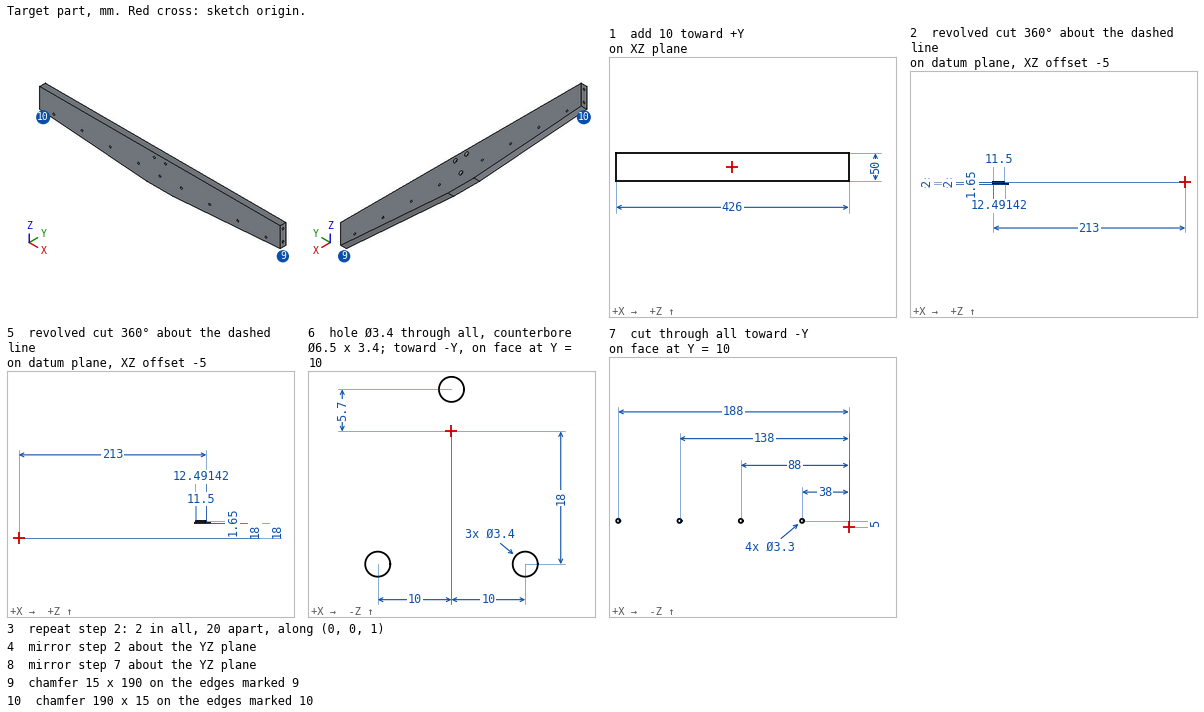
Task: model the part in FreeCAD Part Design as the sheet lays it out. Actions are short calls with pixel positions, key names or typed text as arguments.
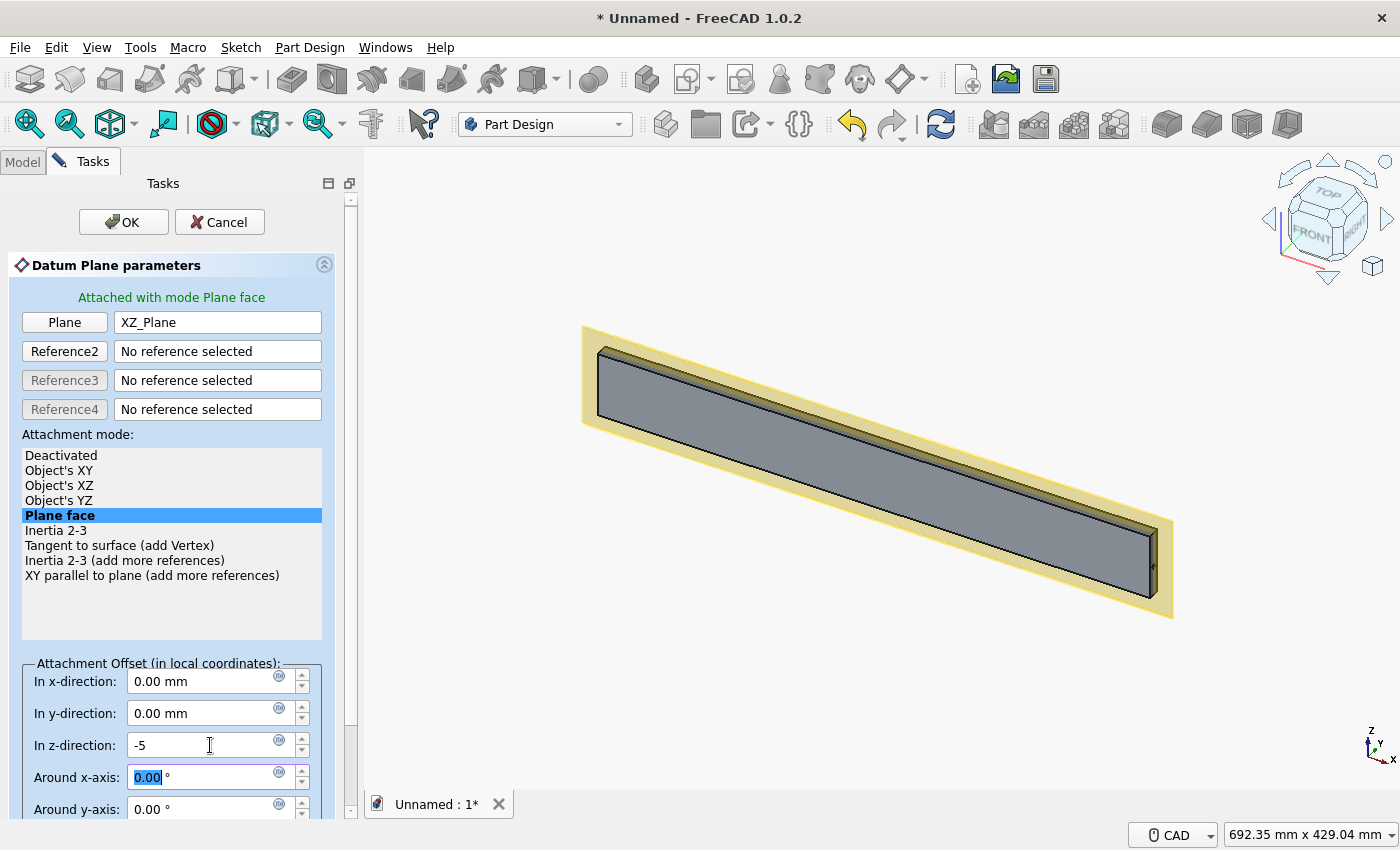
click(124, 222)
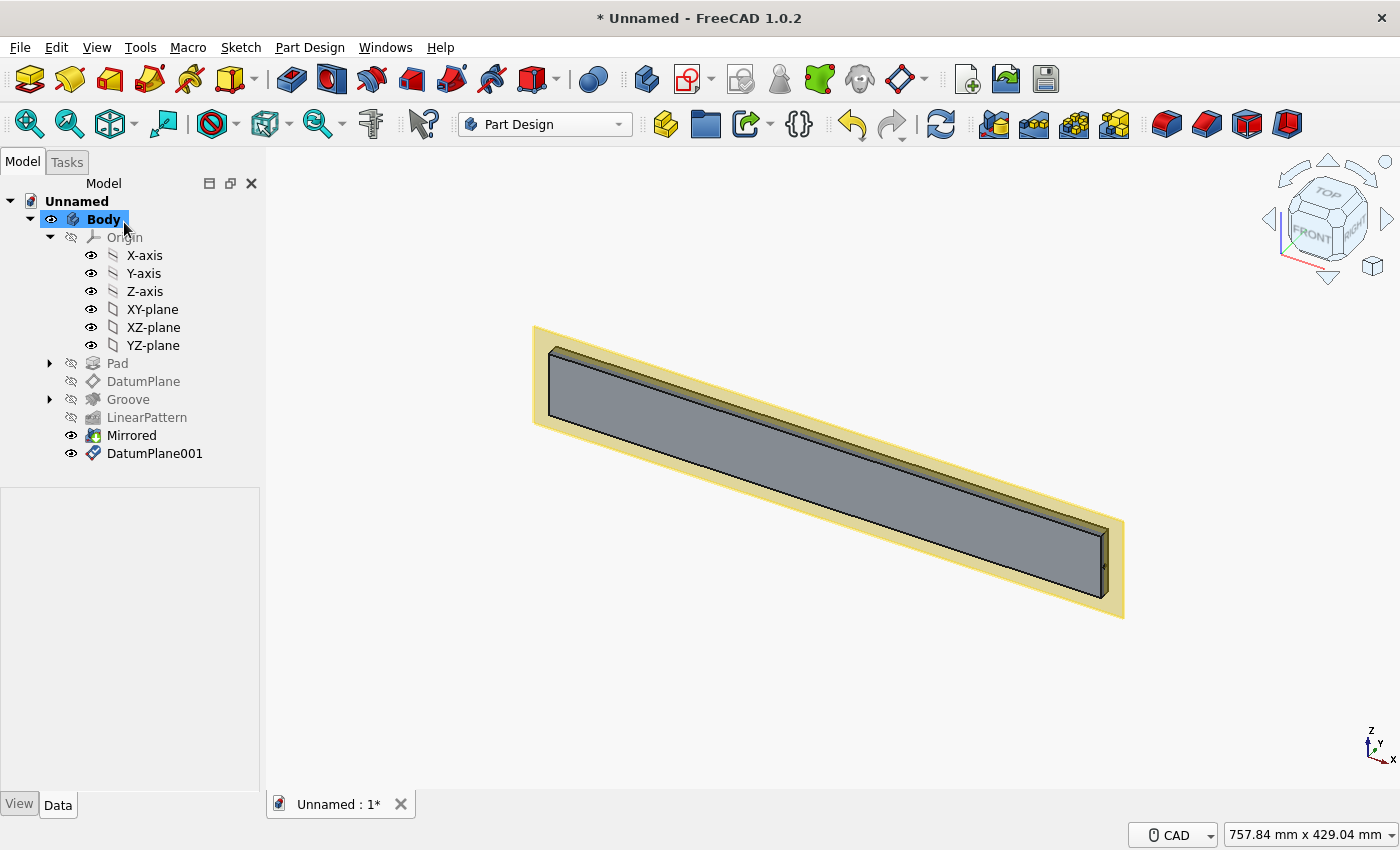
click(116, 453)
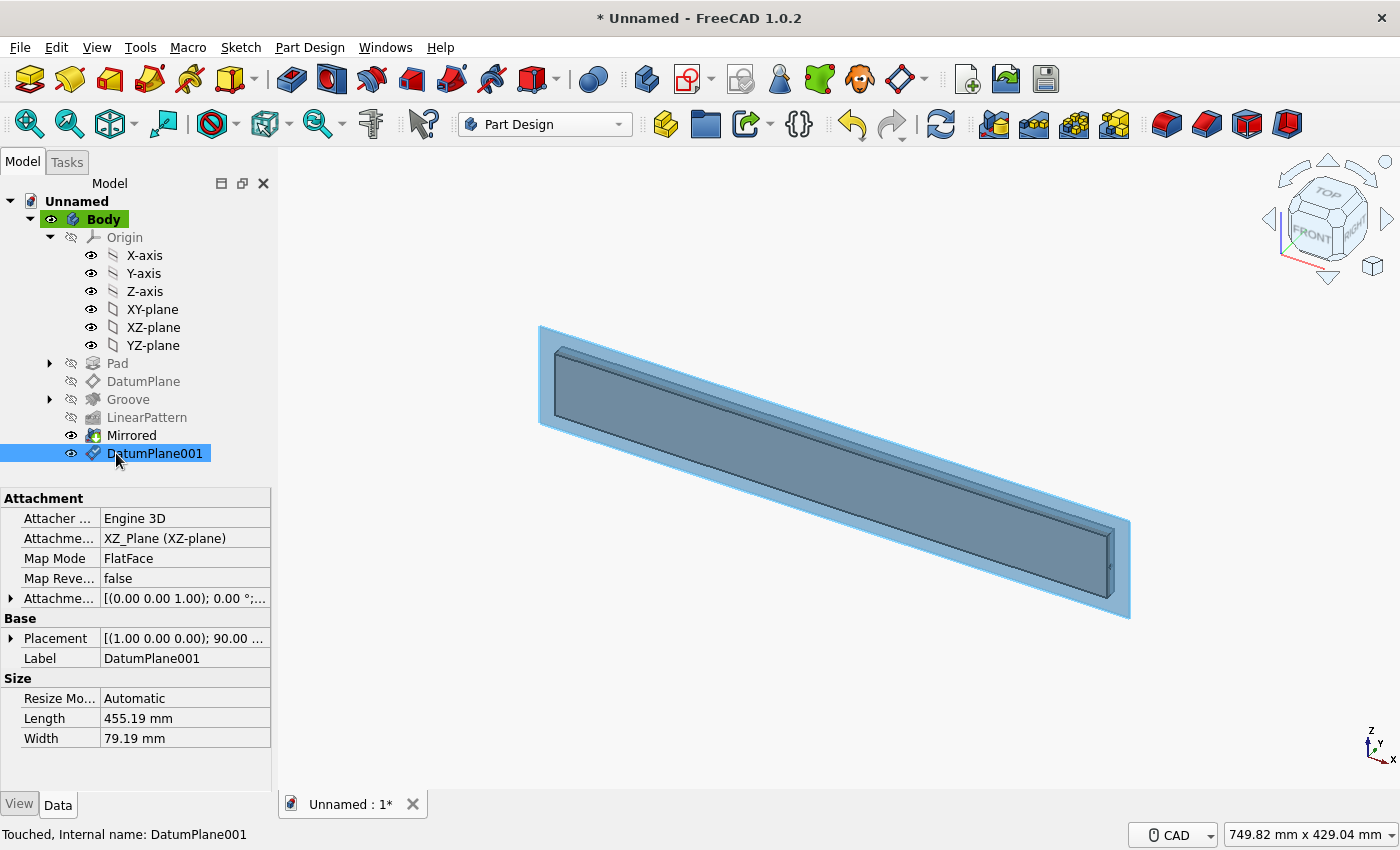
click(688, 80)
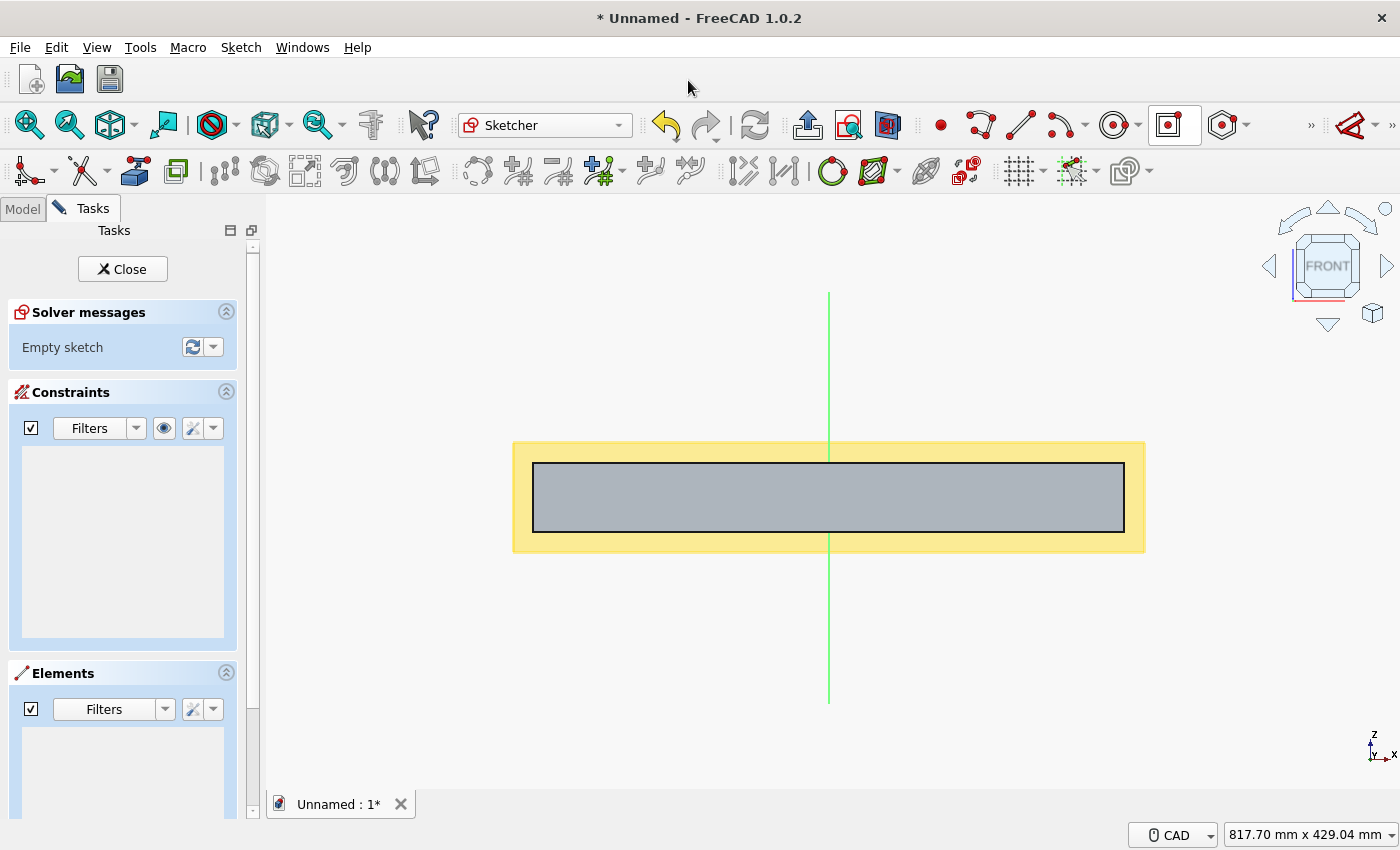
key(q)
key(s)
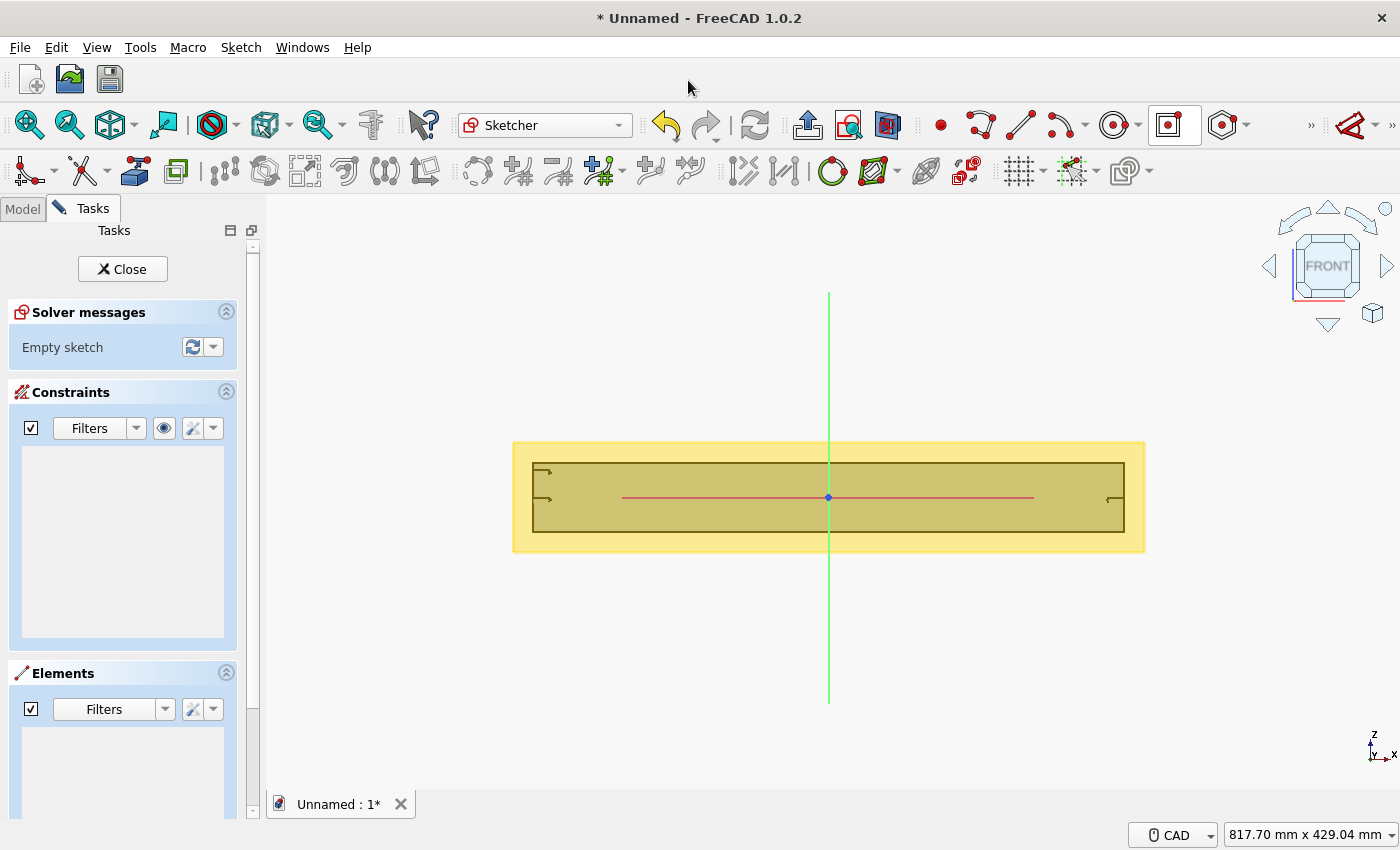
scroll(1137, 470, up, 15)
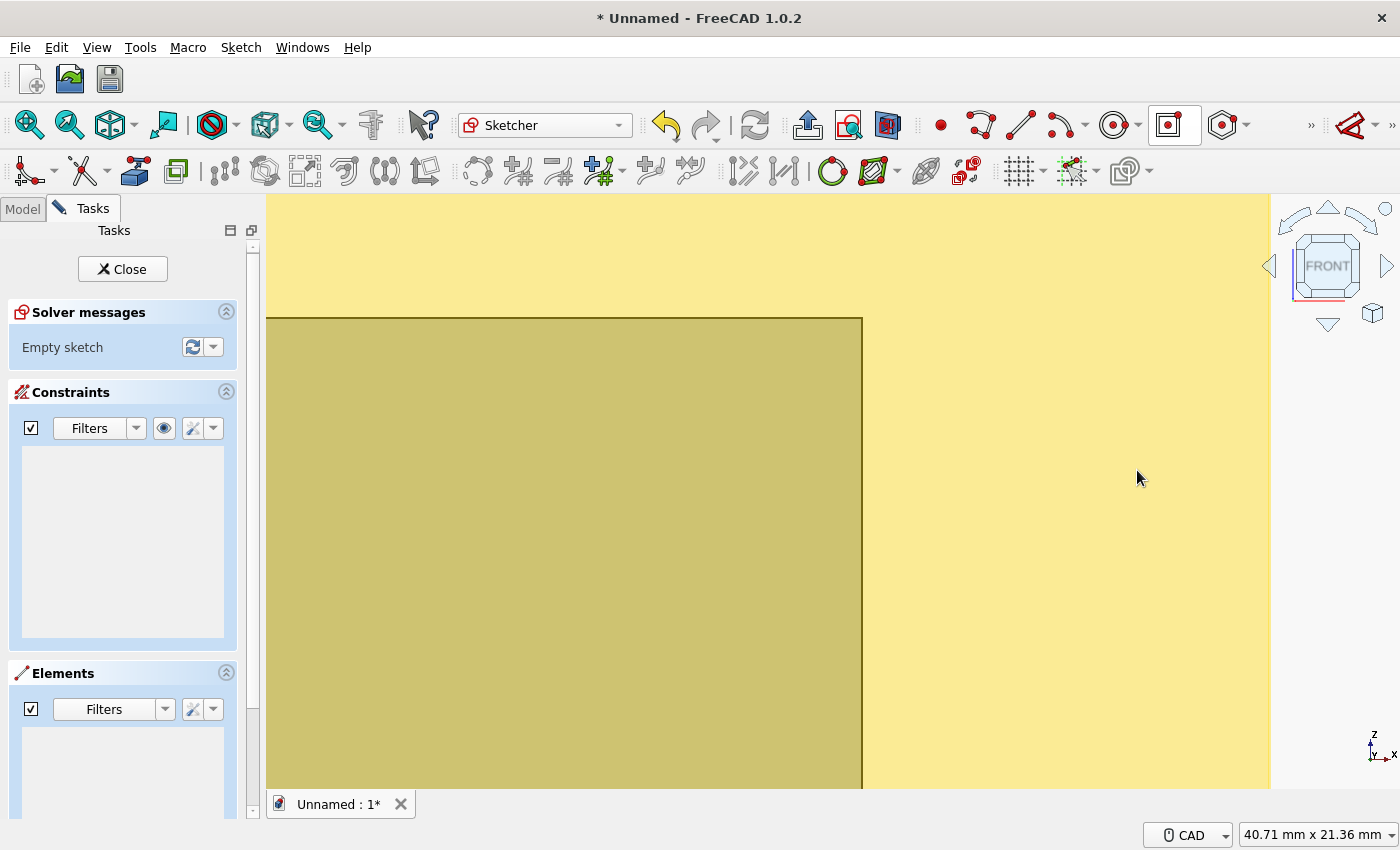
scroll(745, 488, up, 2)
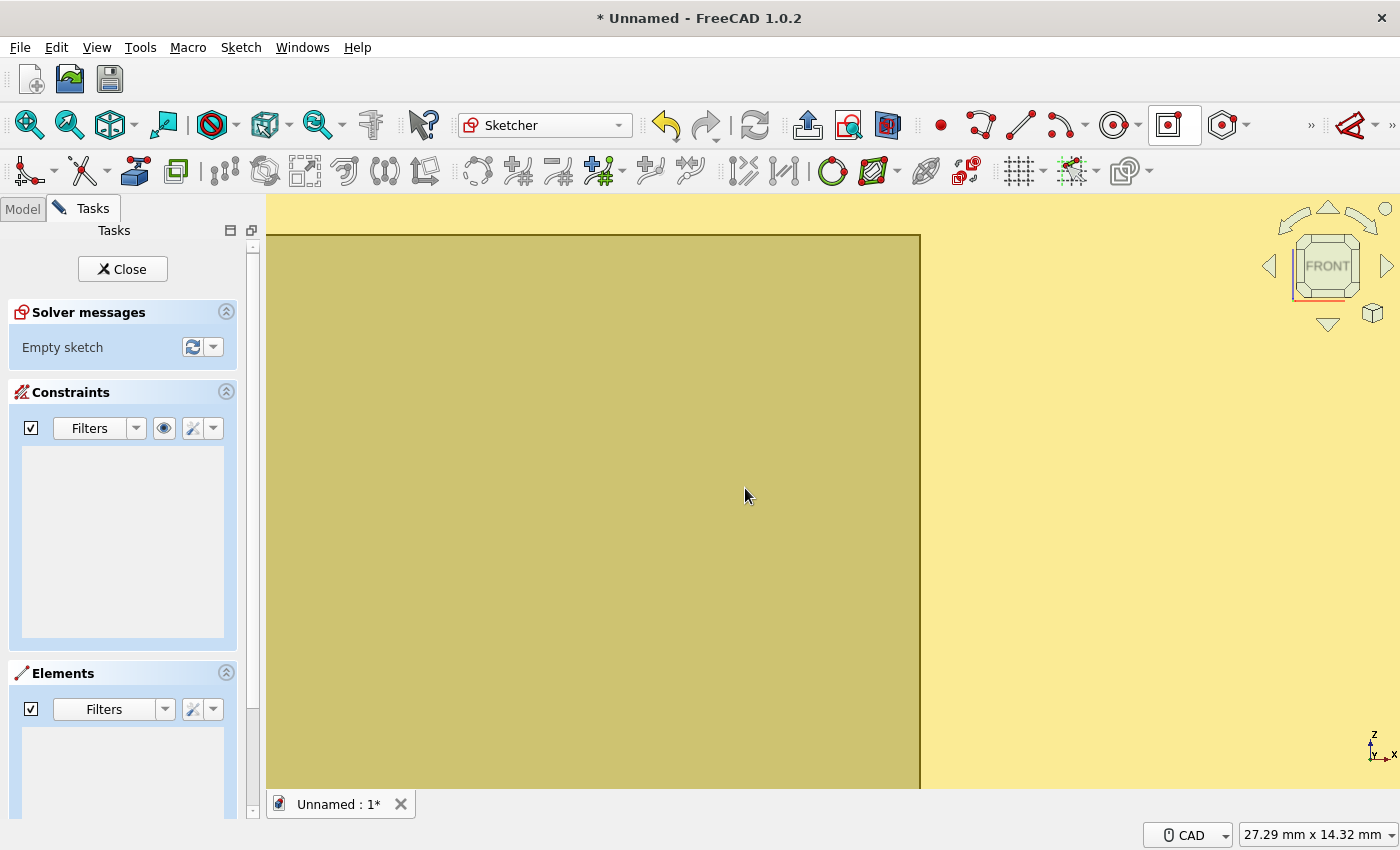
click(982, 126)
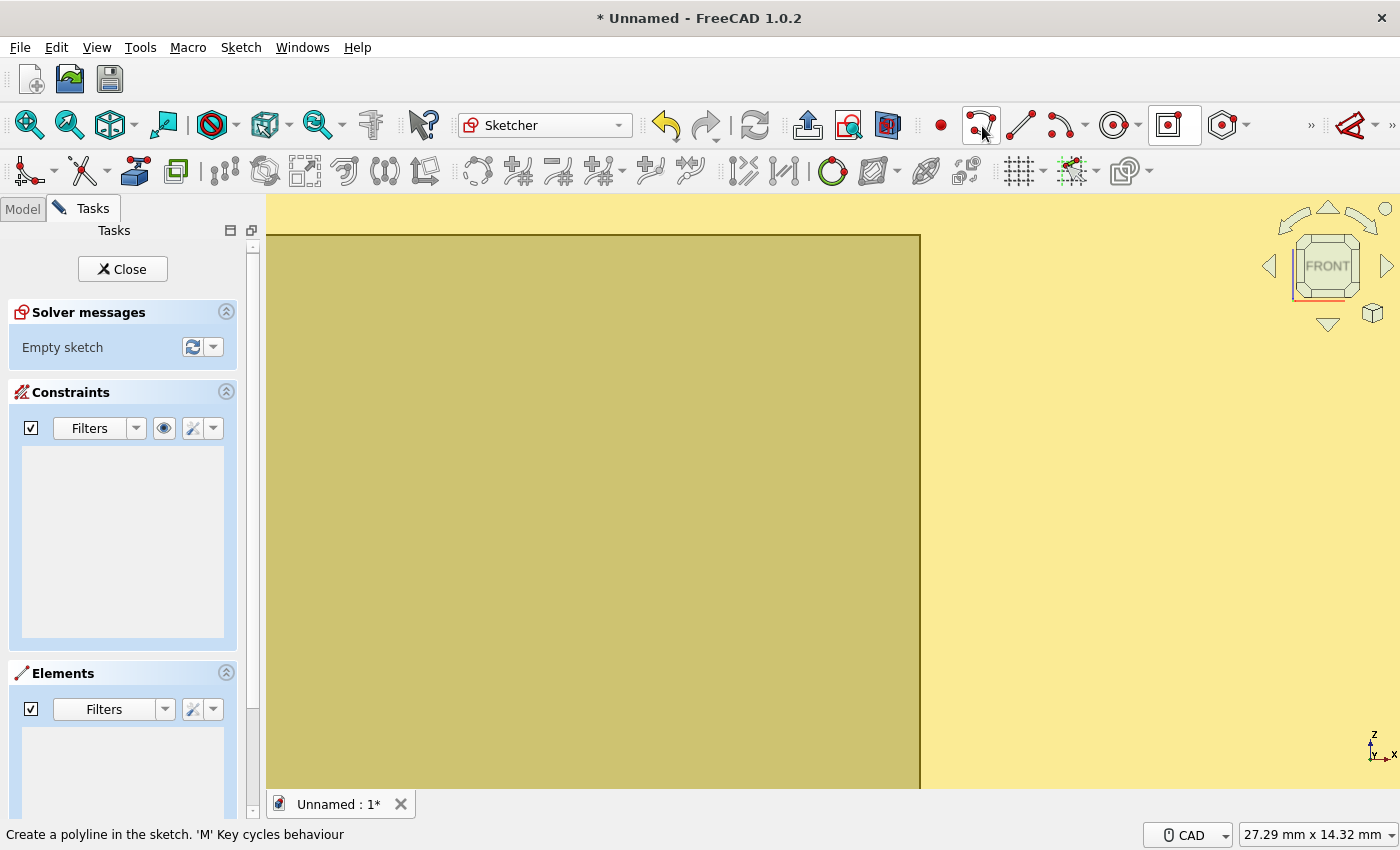
click(401, 526)
click(442, 457)
click(920, 457)
click(920, 526)
click(401, 527)